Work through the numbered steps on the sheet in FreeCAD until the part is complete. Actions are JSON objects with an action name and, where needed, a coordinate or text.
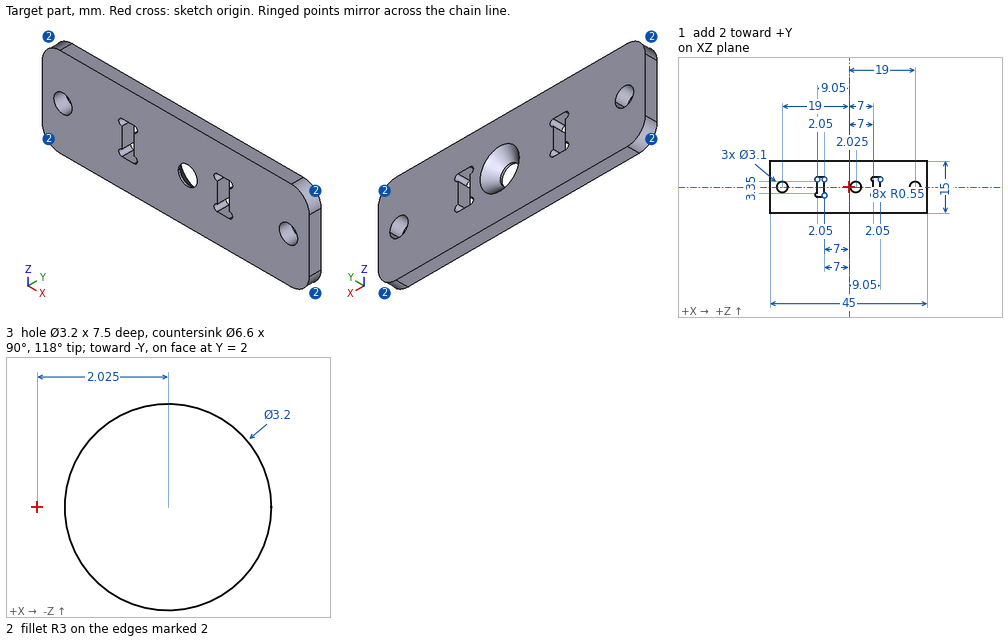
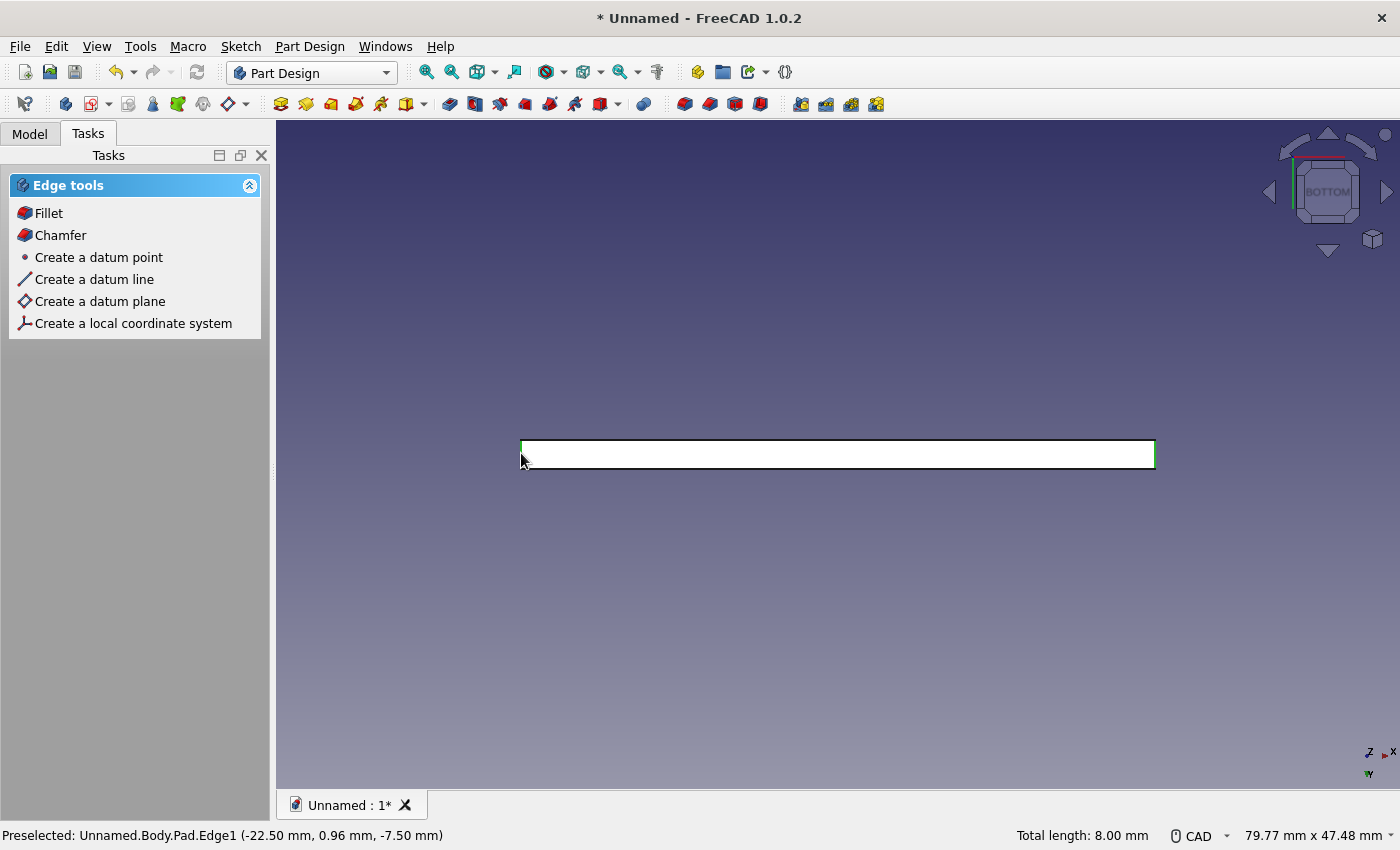
{"action": "left_click", "coordinate": [685, 104]}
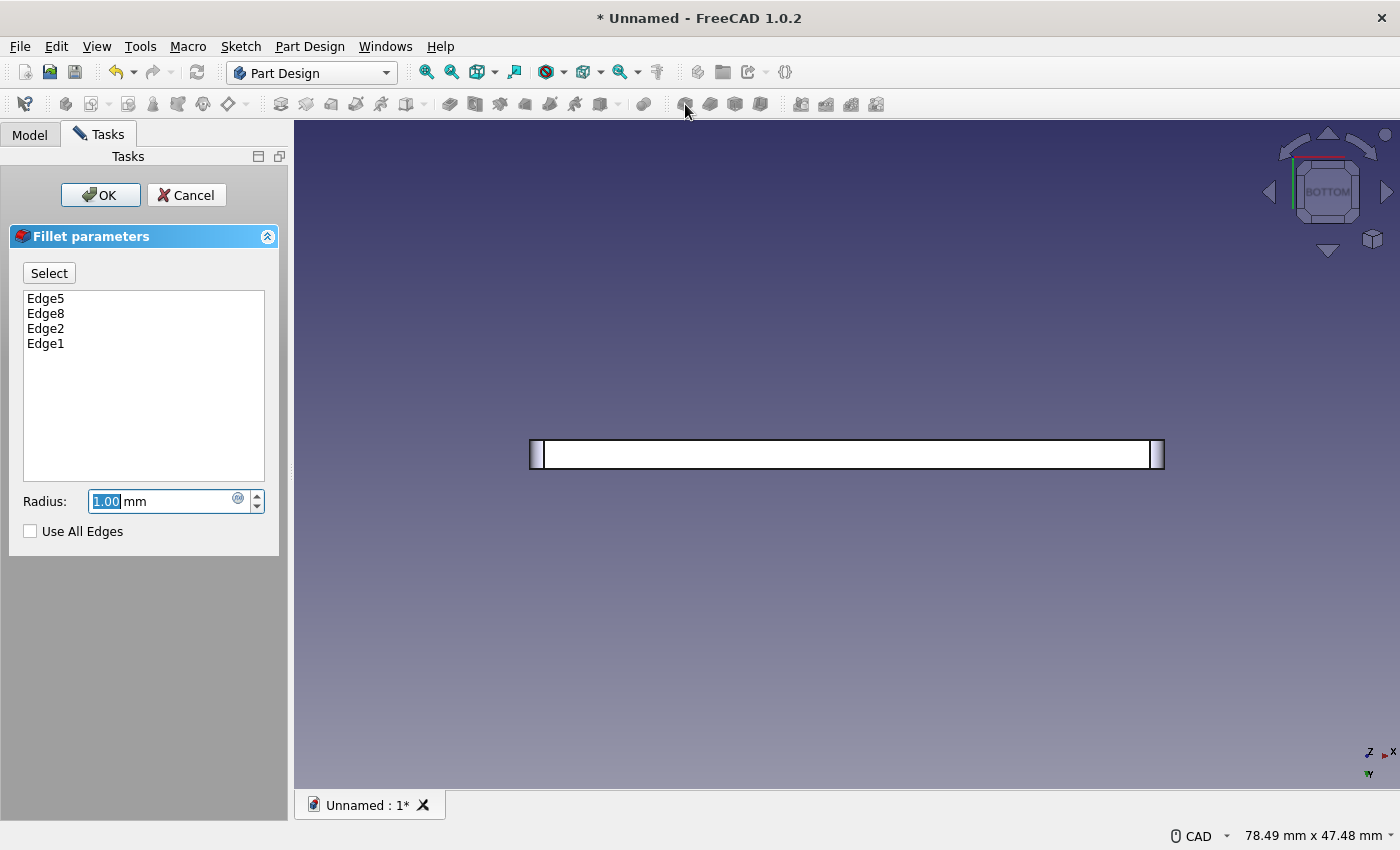
{"action": "type", "text": "3"}
{"action": "key", "text": "Tab"}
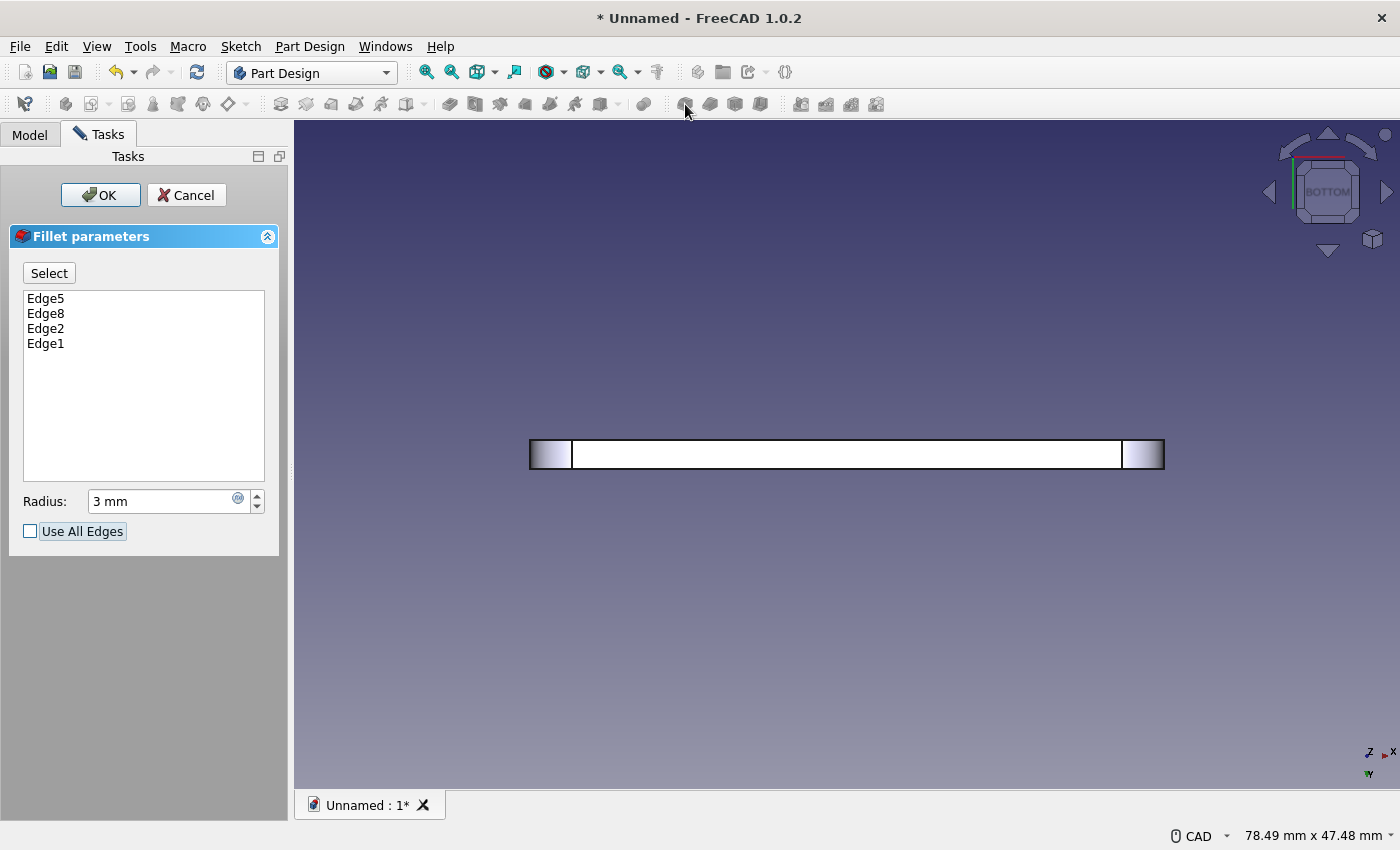
{"action": "left_click", "coordinate": [101, 195]}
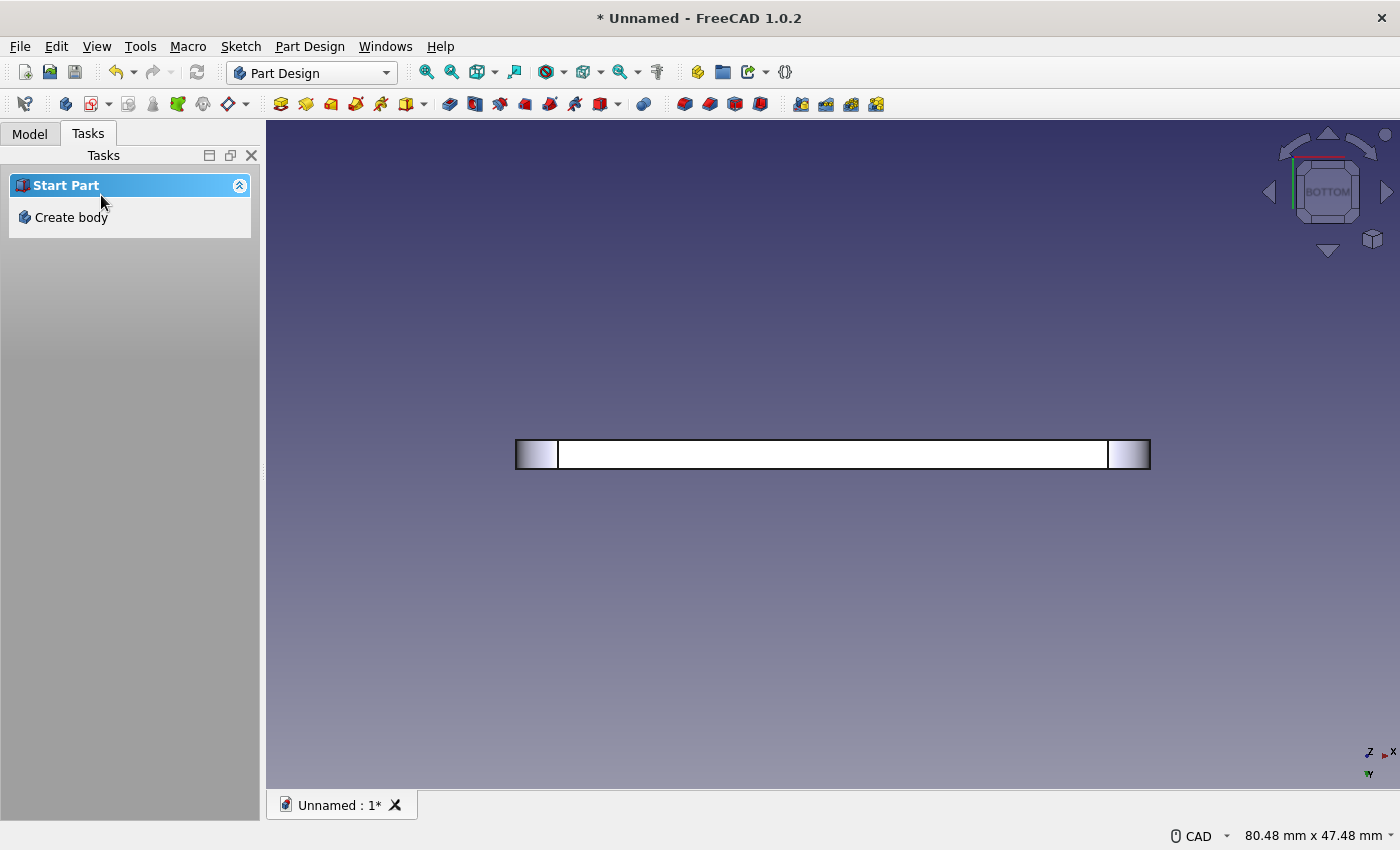
{"action": "key", "text": "4"}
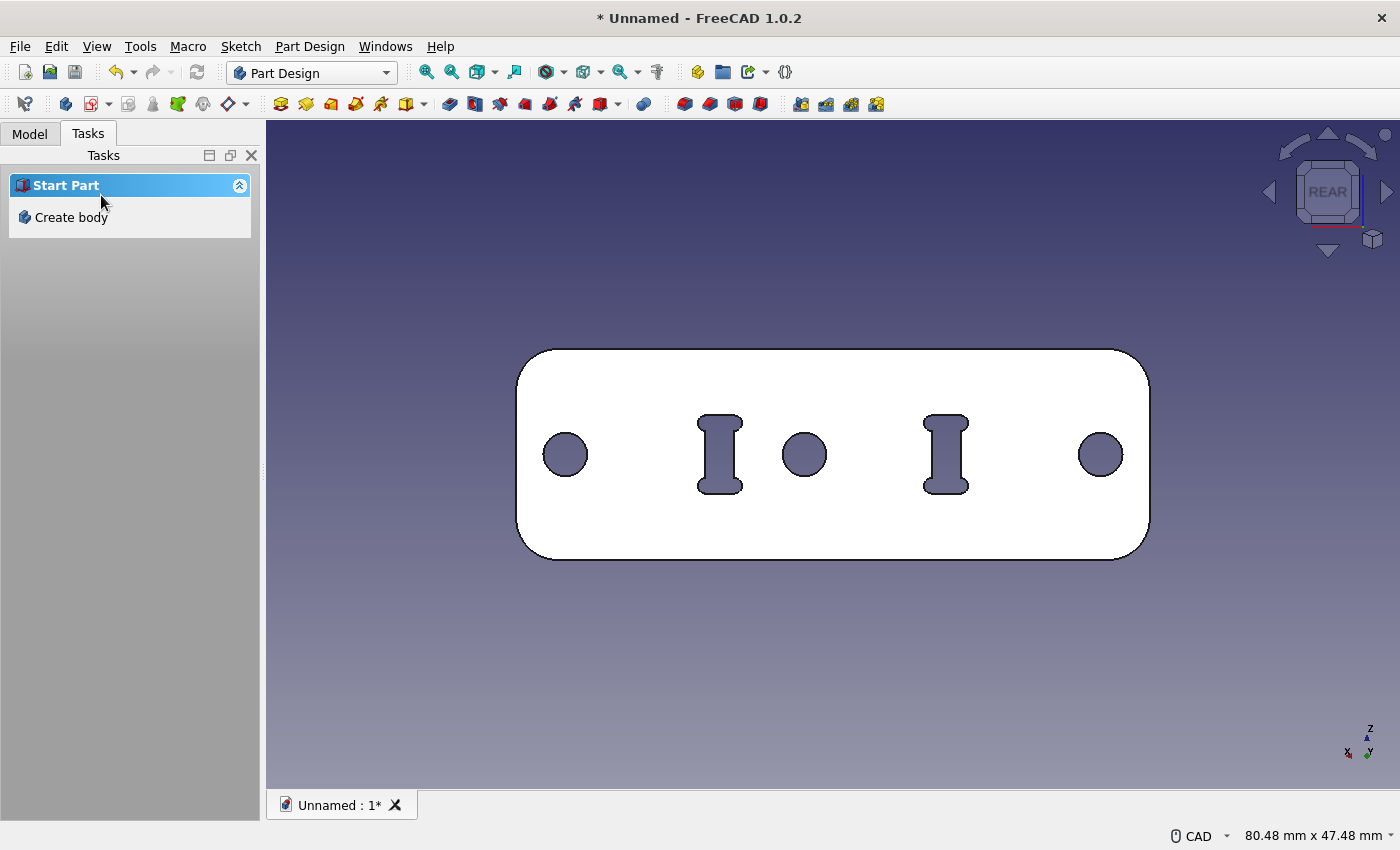
{"action": "left_click", "coordinate": [1014, 454]}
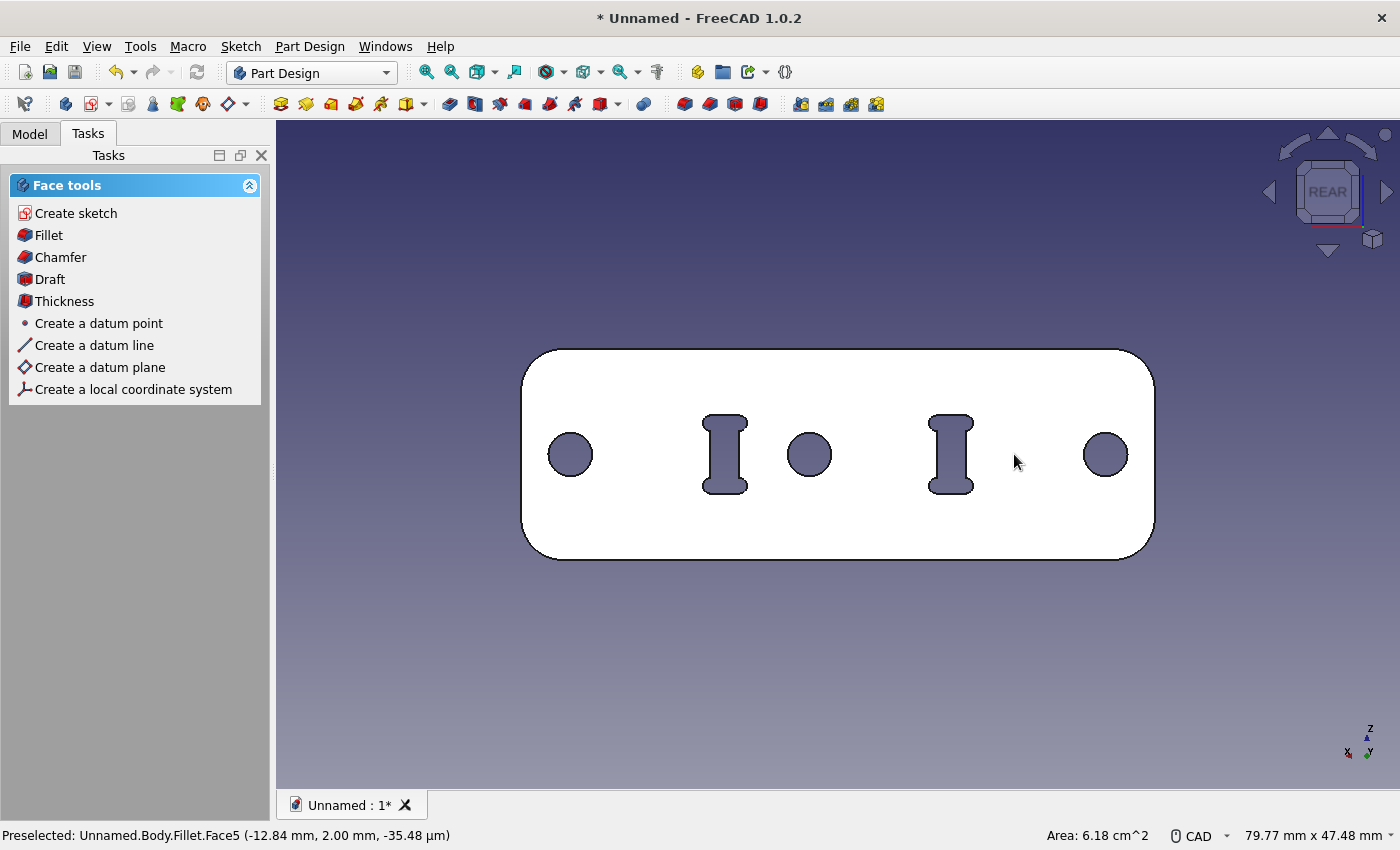
{"action": "left_click", "coordinate": [90, 104]}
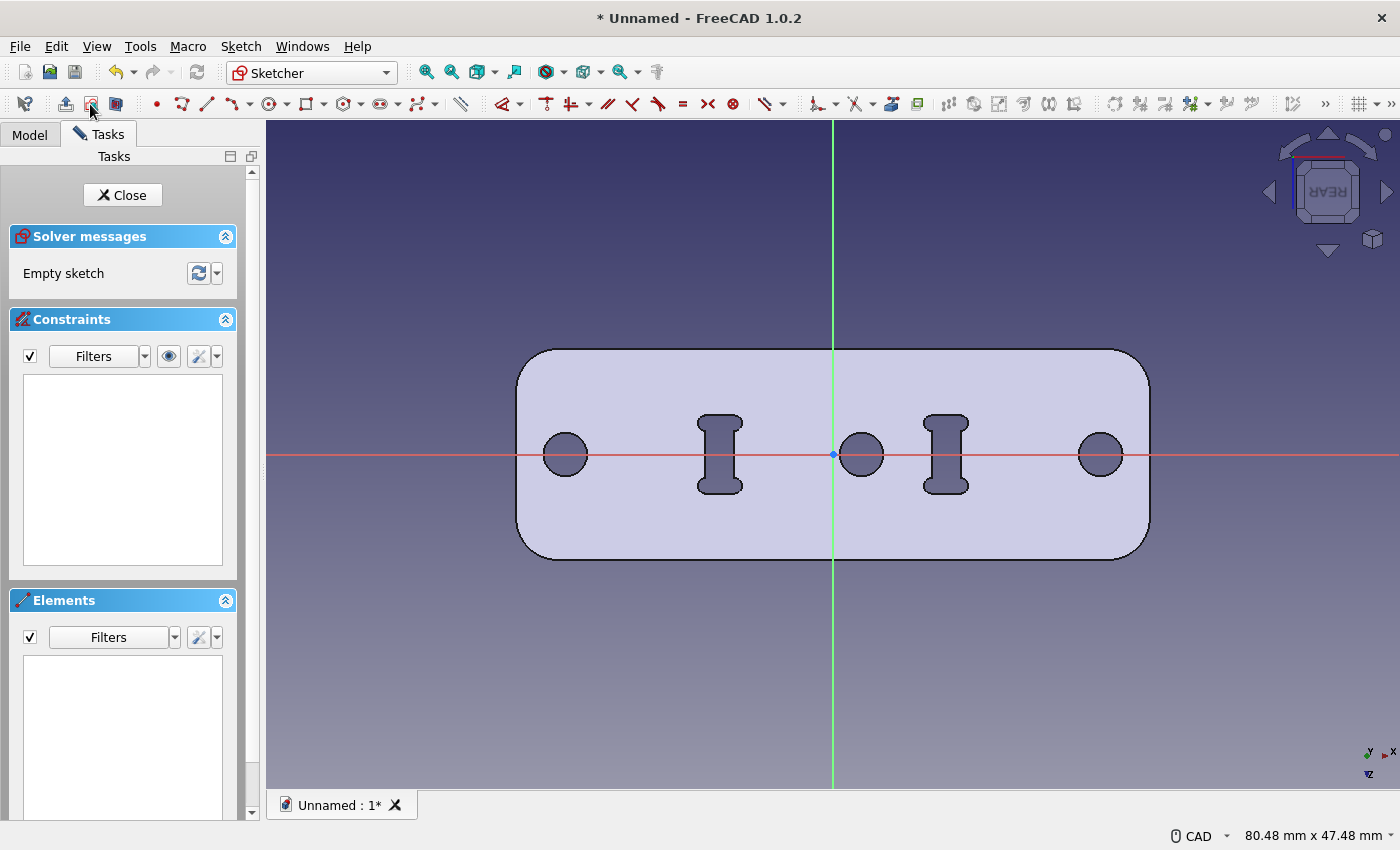
{"action": "scroll", "coordinate": [870, 454], "scroll_direction": "up", "scroll_amount": 11}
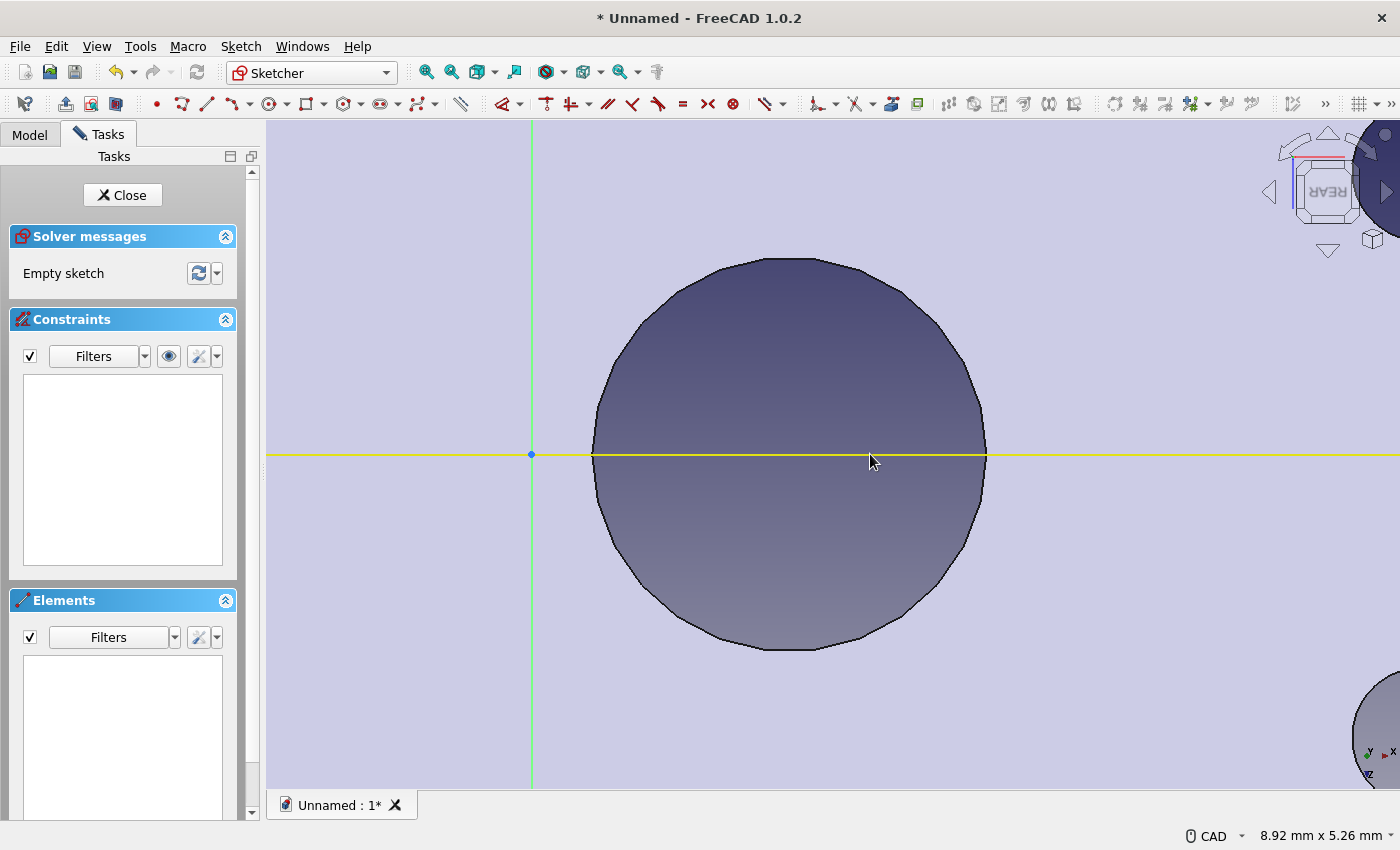
{"action": "left_click", "coordinate": [268, 104]}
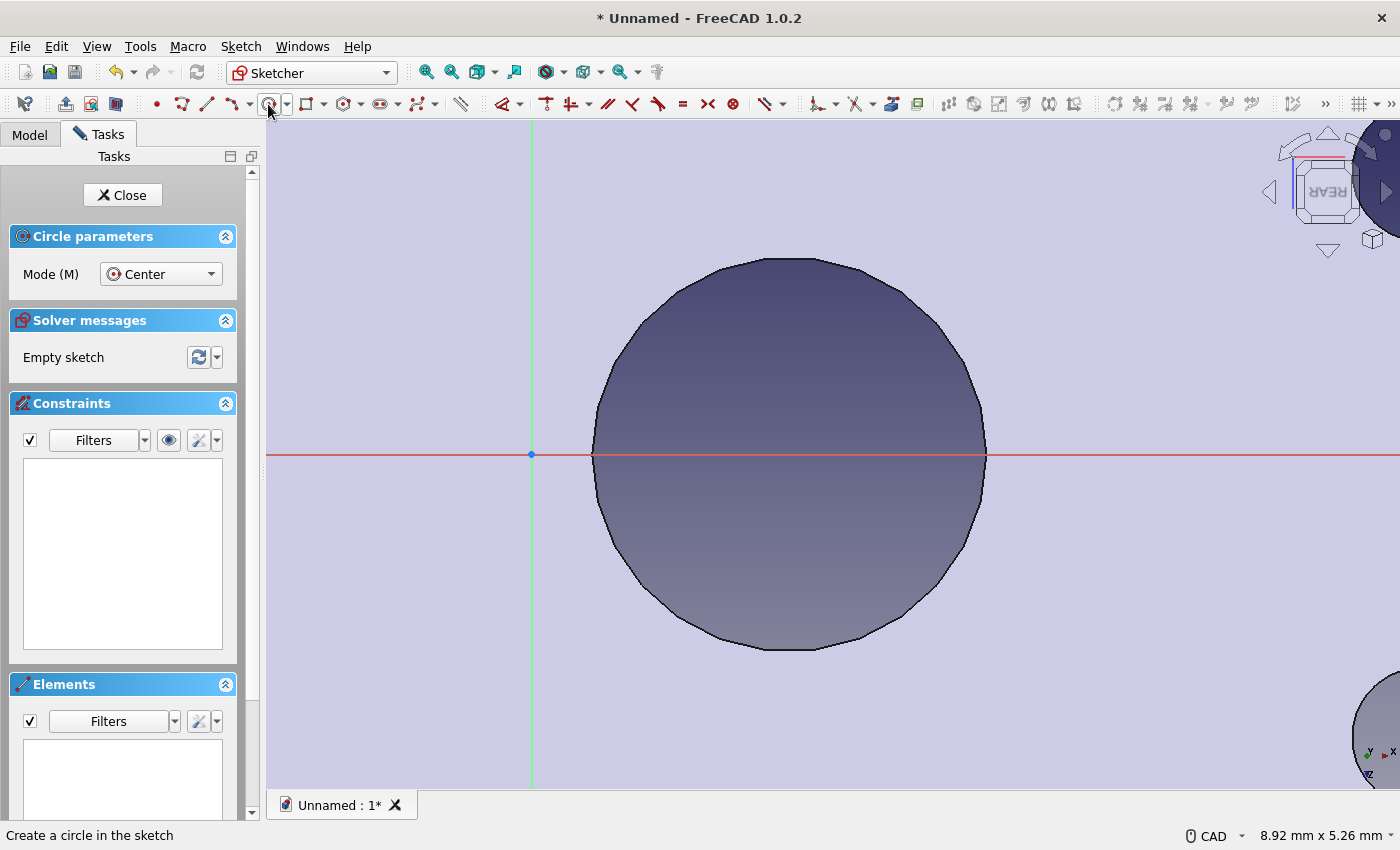
{"action": "left_click", "coordinate": [789, 454]}
{"action": "mouse_move", "coordinate": [933, 311]}